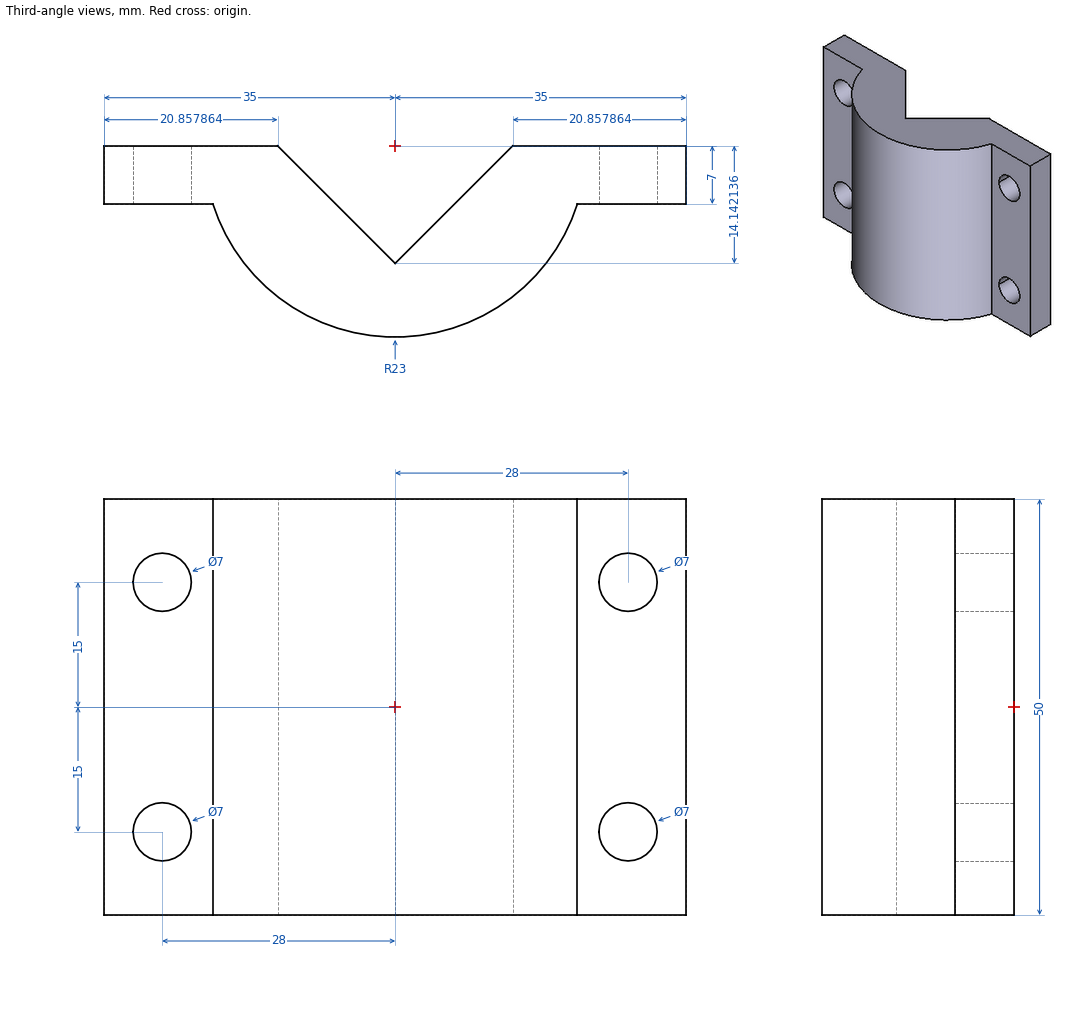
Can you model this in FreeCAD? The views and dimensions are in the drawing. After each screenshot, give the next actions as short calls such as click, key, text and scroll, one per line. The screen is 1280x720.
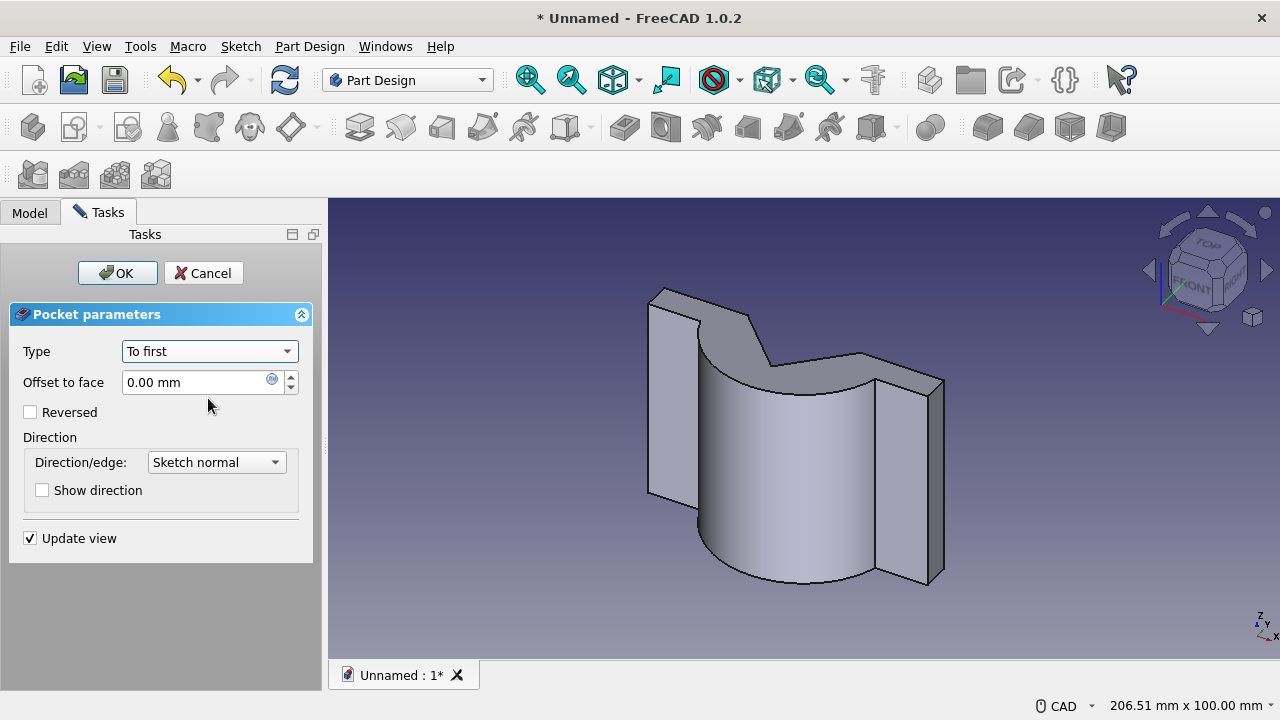
click(31, 412)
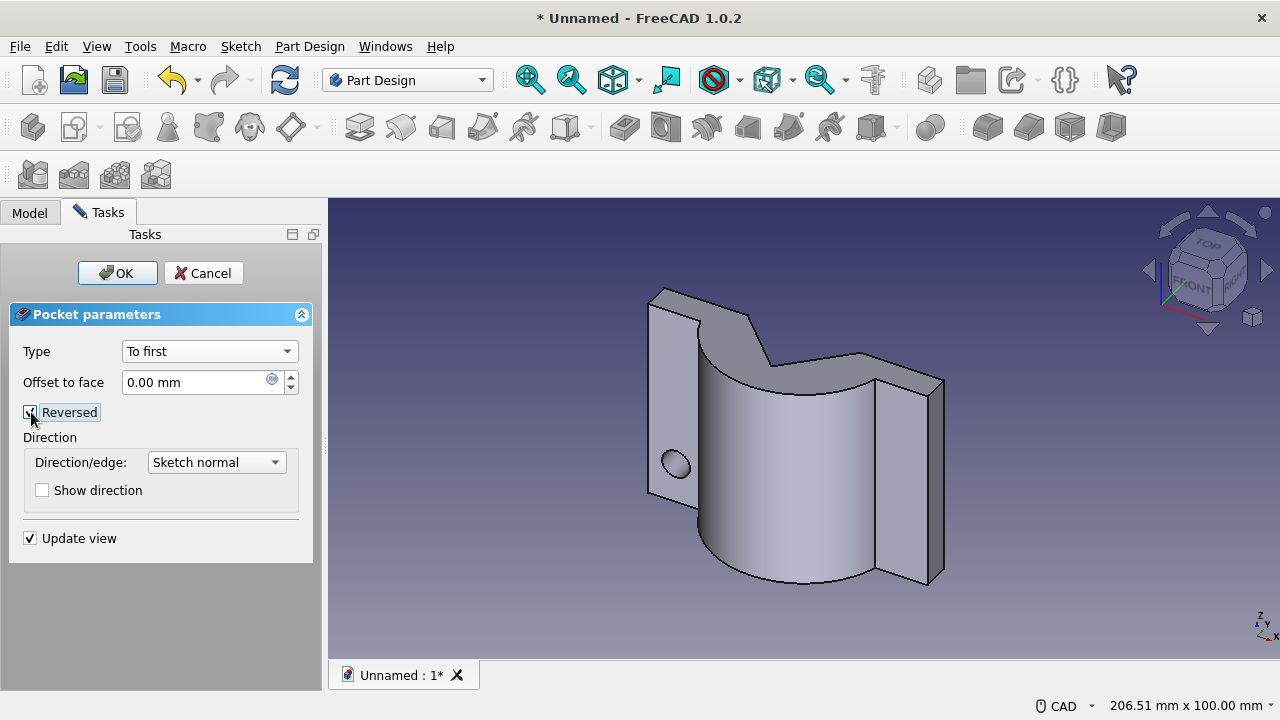
click(118, 273)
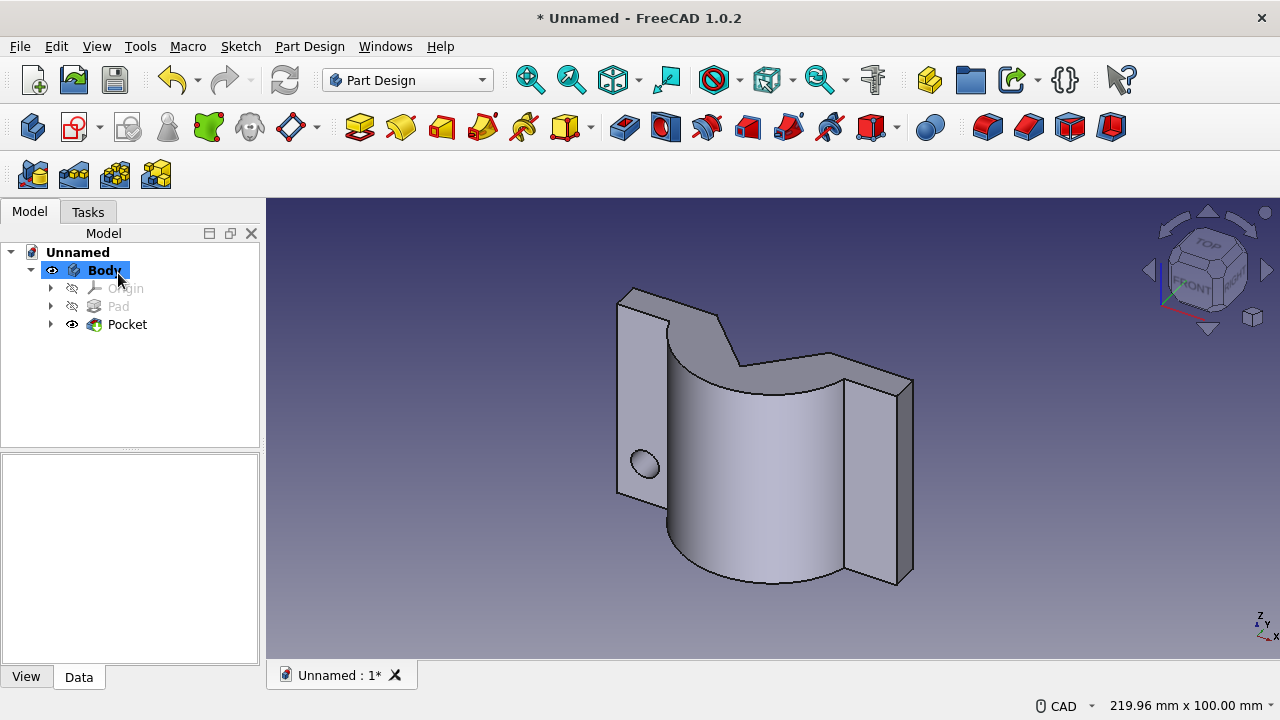
click(74, 128)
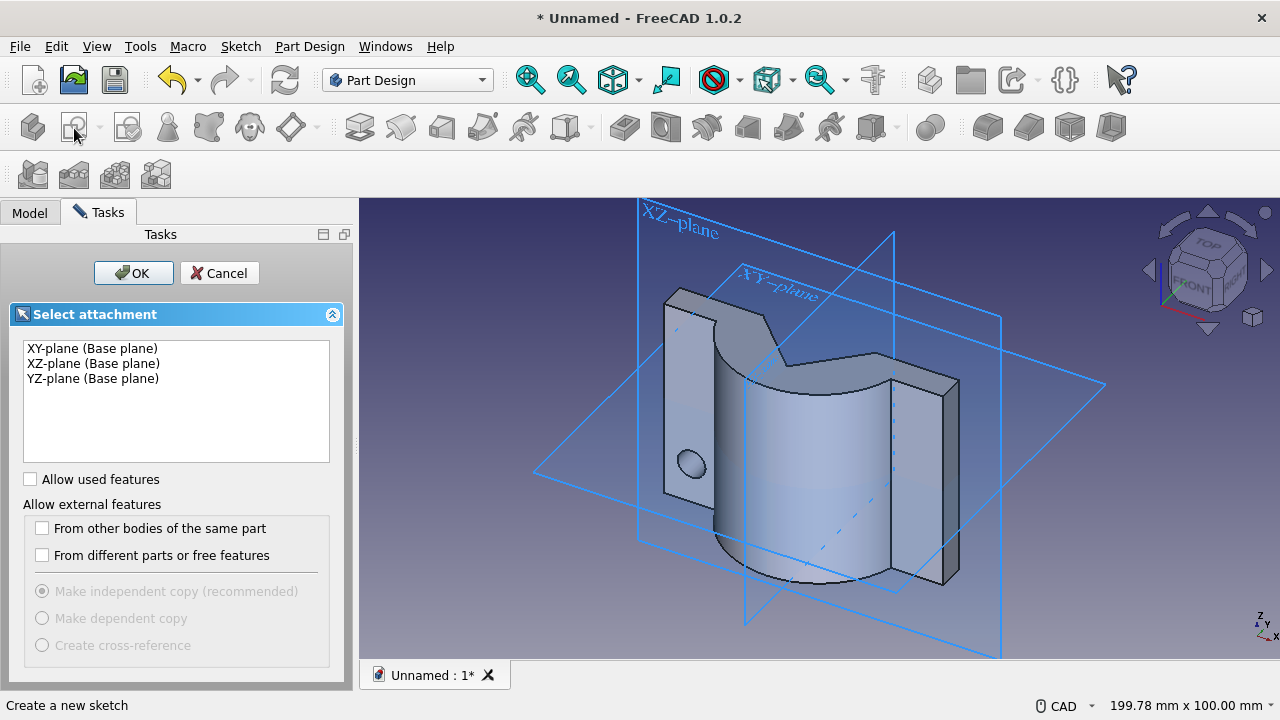
click(84, 364)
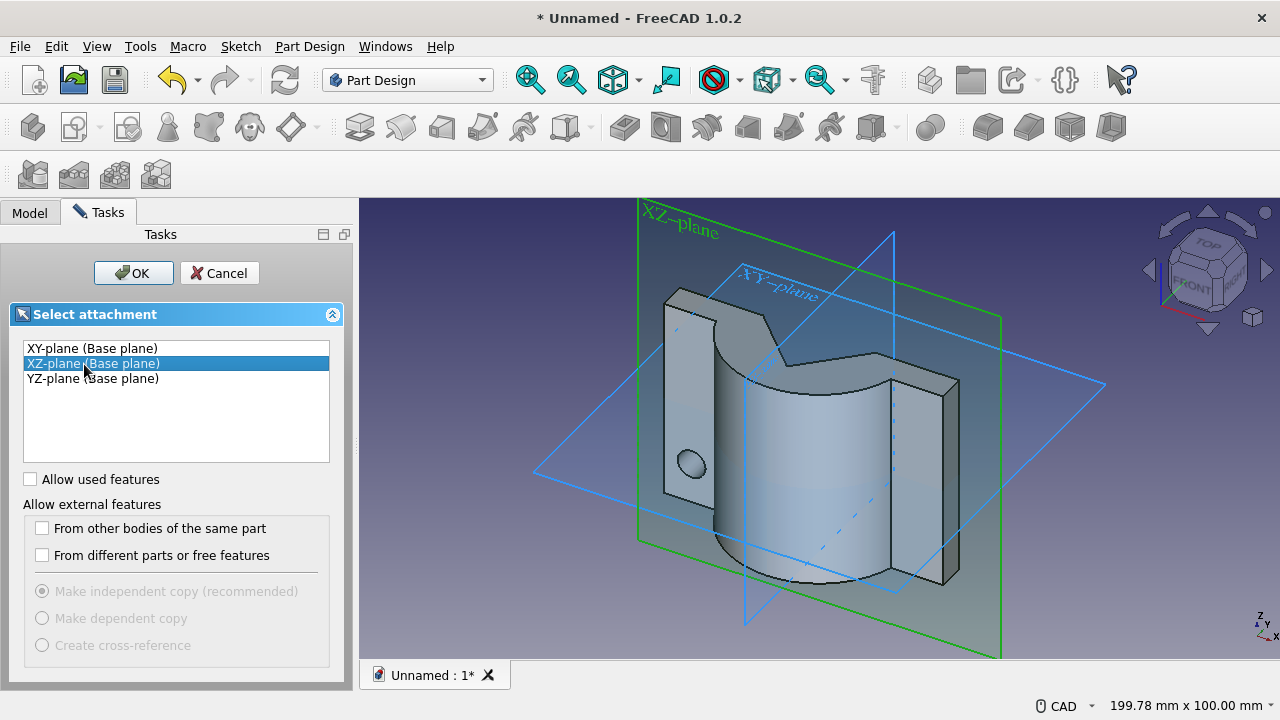
click(134, 273)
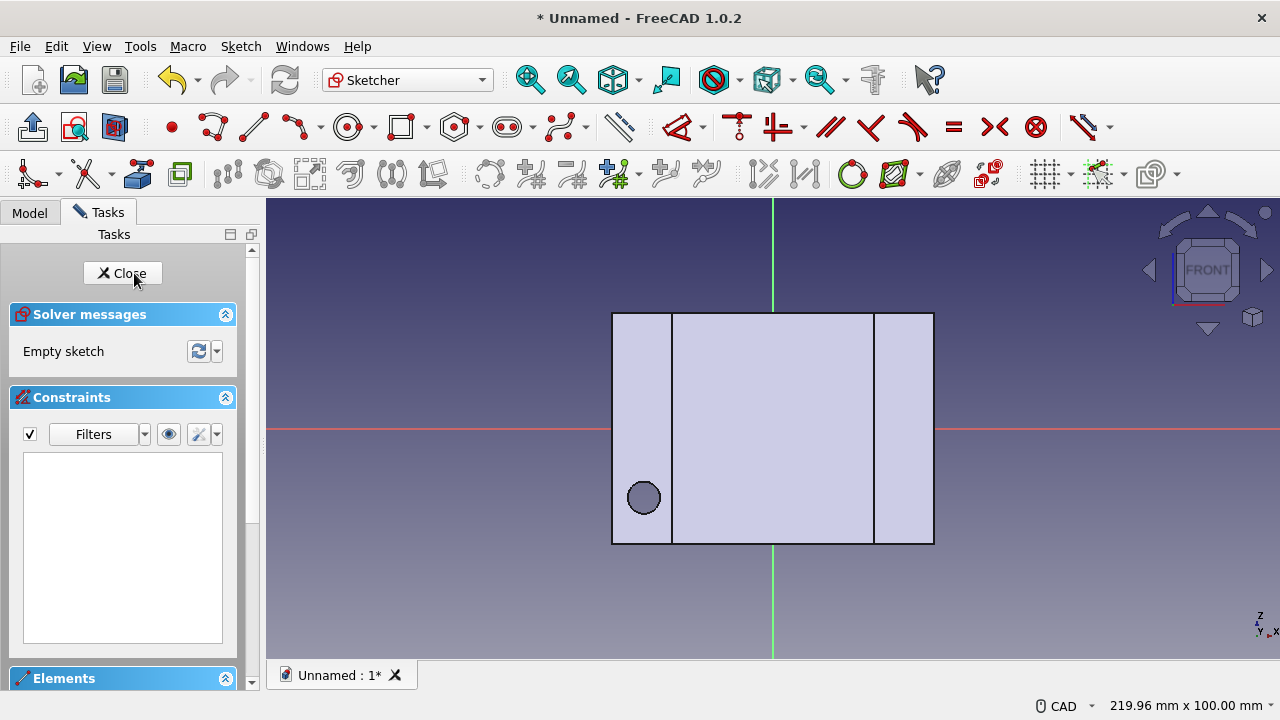
key(q)
key(s)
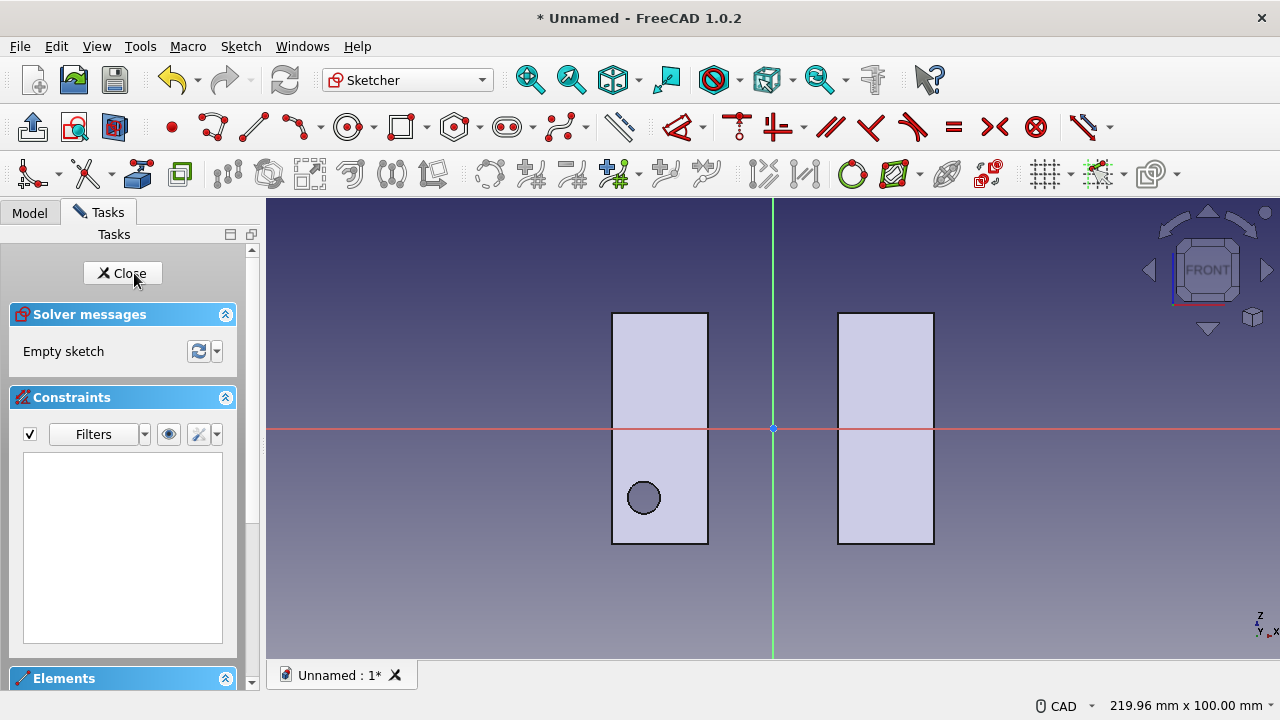
scroll(636, 351, up, 11)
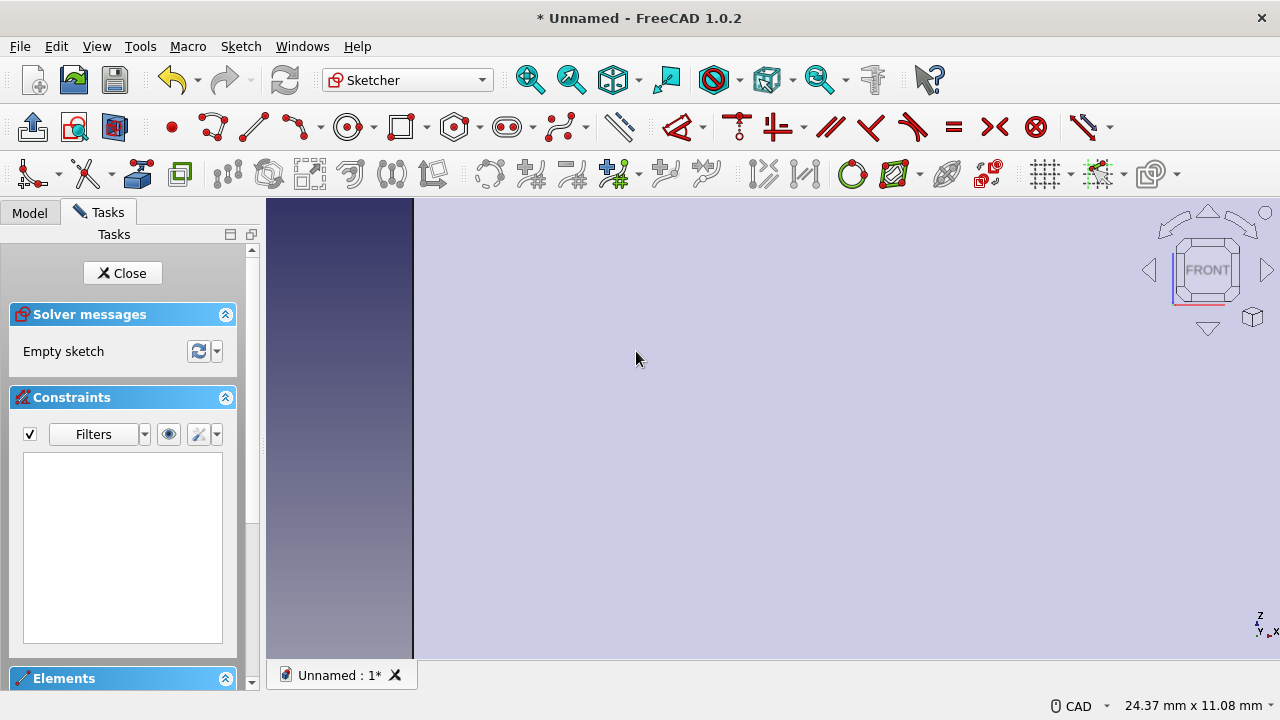
click(348, 128)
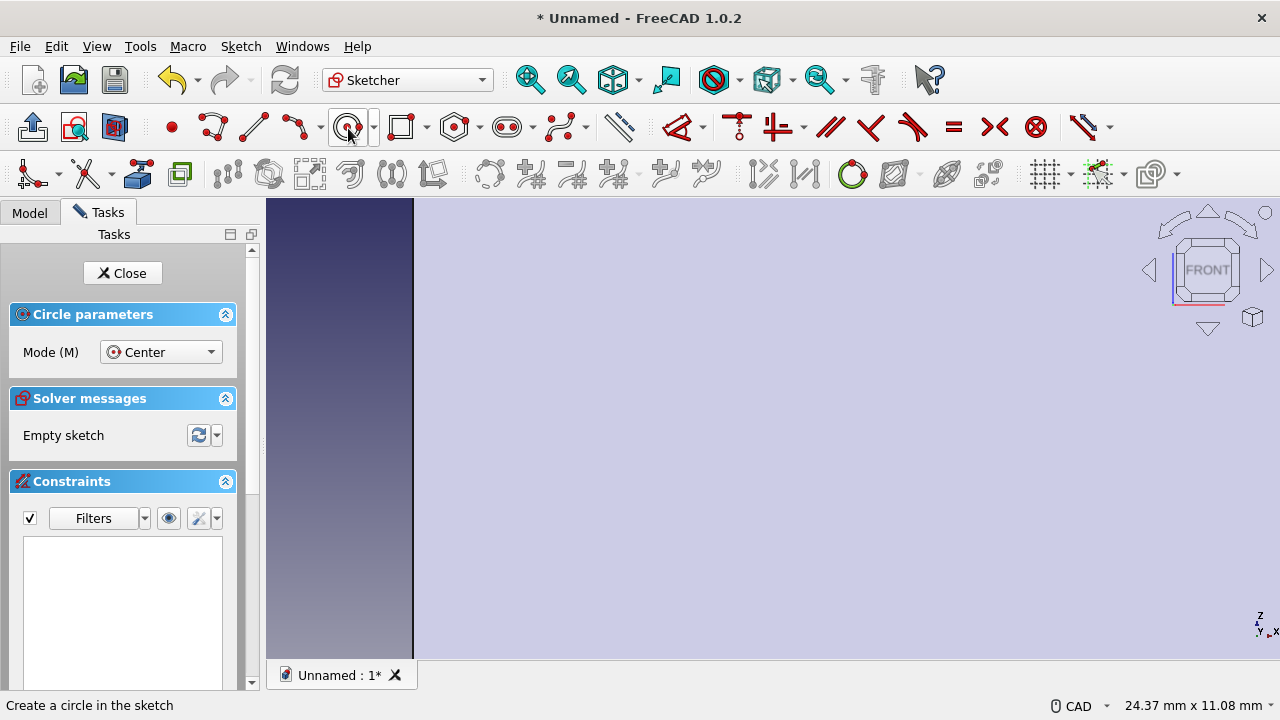
click(705, 424)
click(808, 321)
key(Escape)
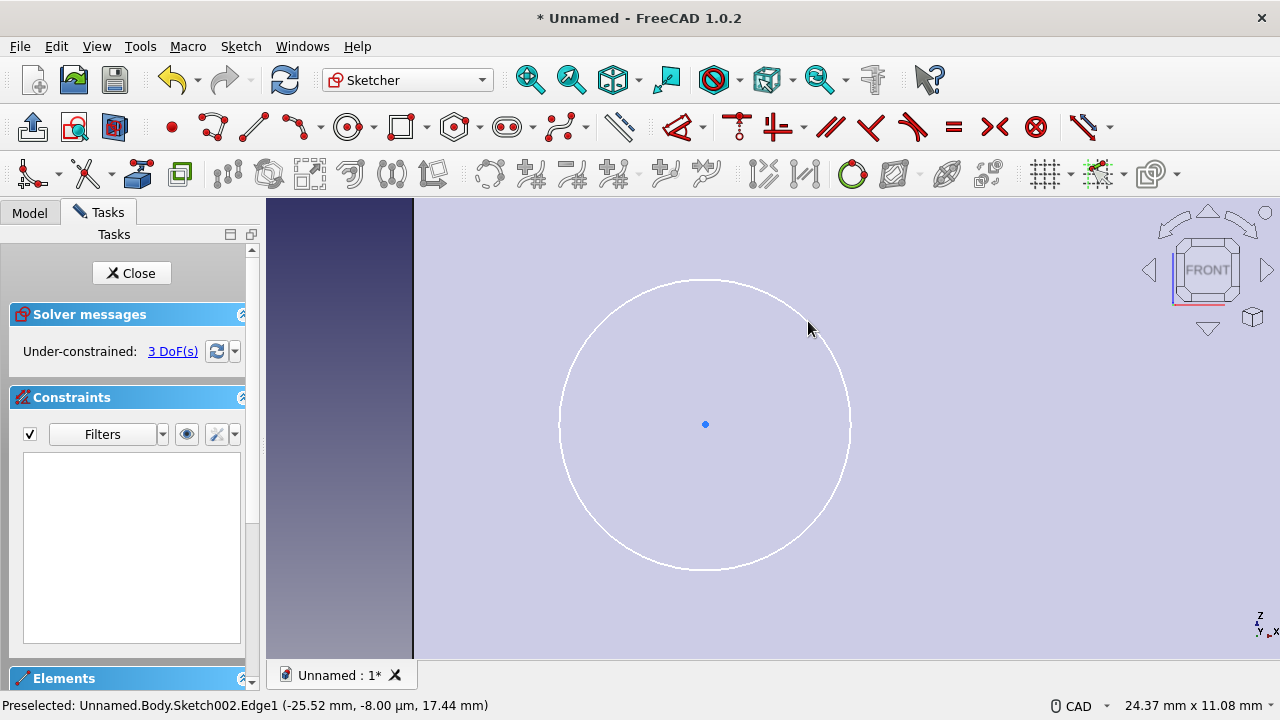
key(d)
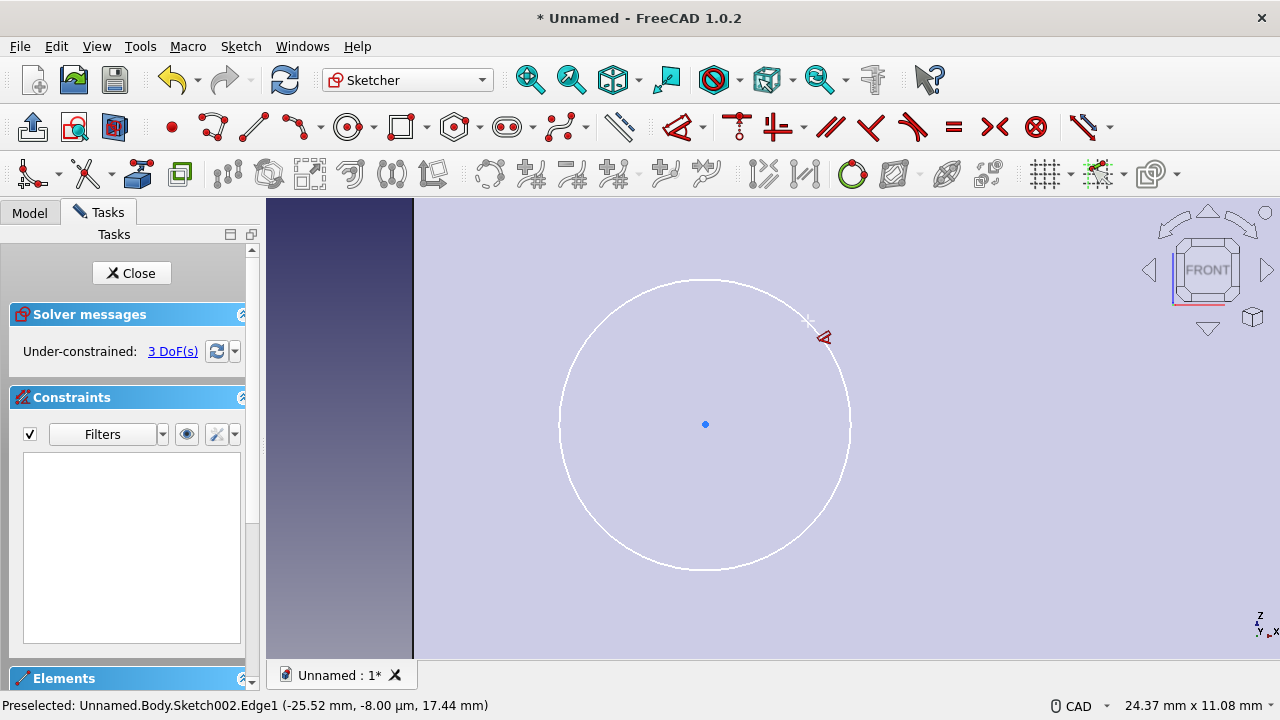
click(808, 322)
click(831, 299)